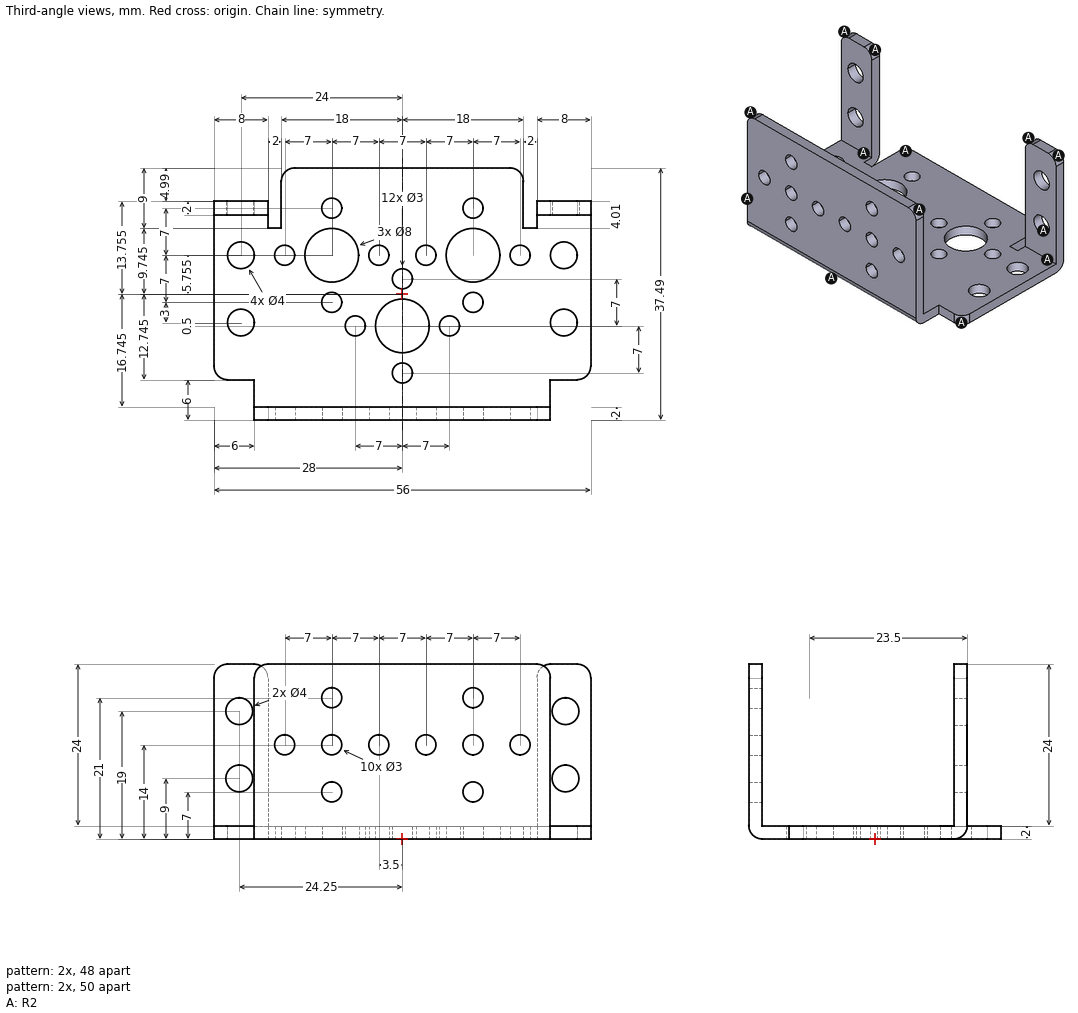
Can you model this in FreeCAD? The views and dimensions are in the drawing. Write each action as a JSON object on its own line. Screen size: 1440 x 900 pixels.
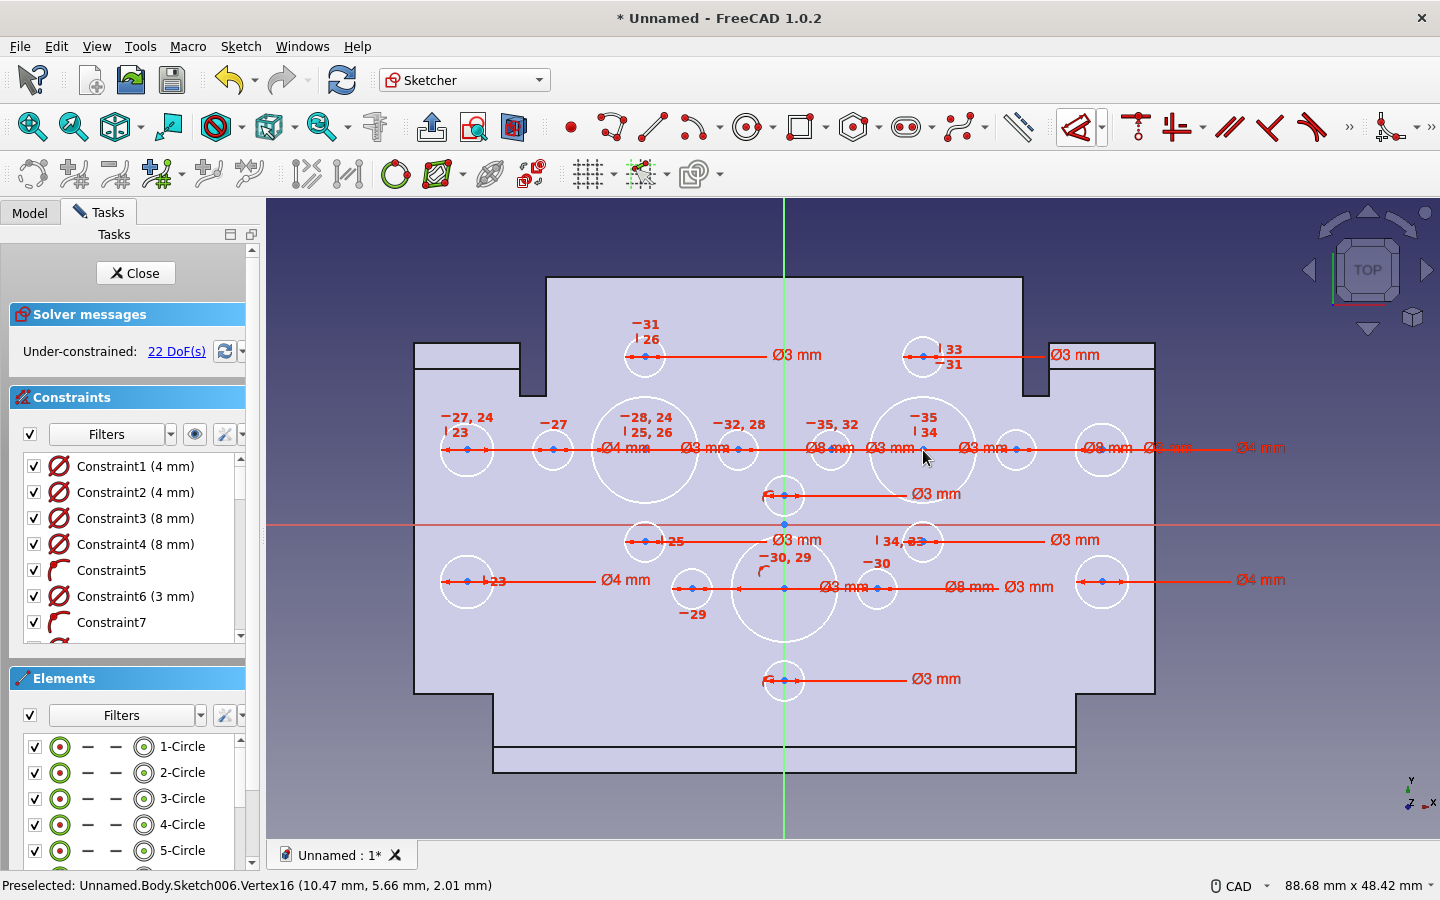
{"action": "left_click", "coordinate": [923, 450]}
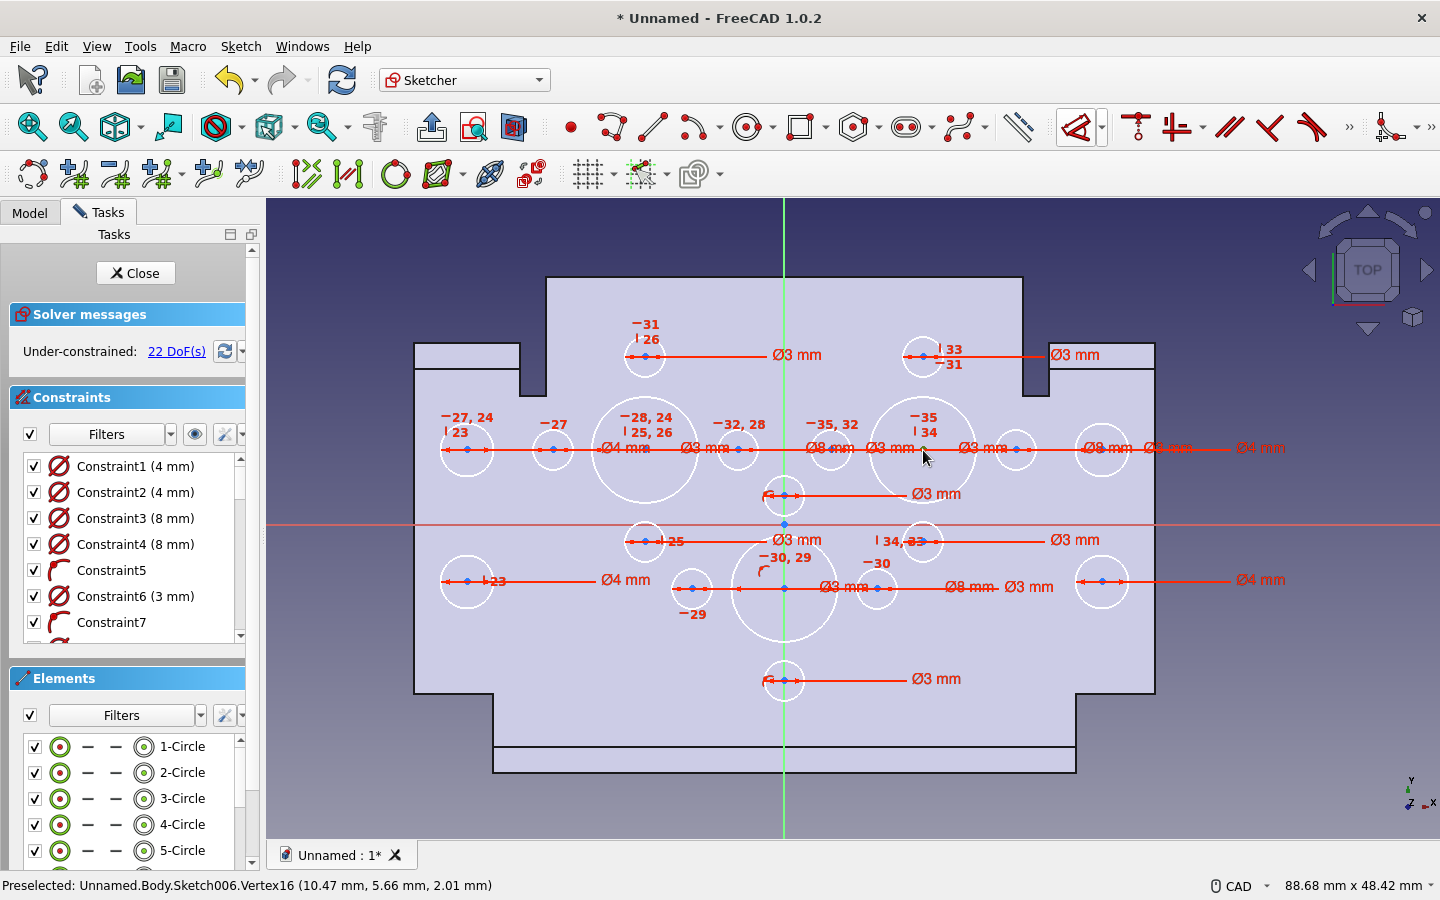
{"action": "left_click", "coordinate": [1016, 450]}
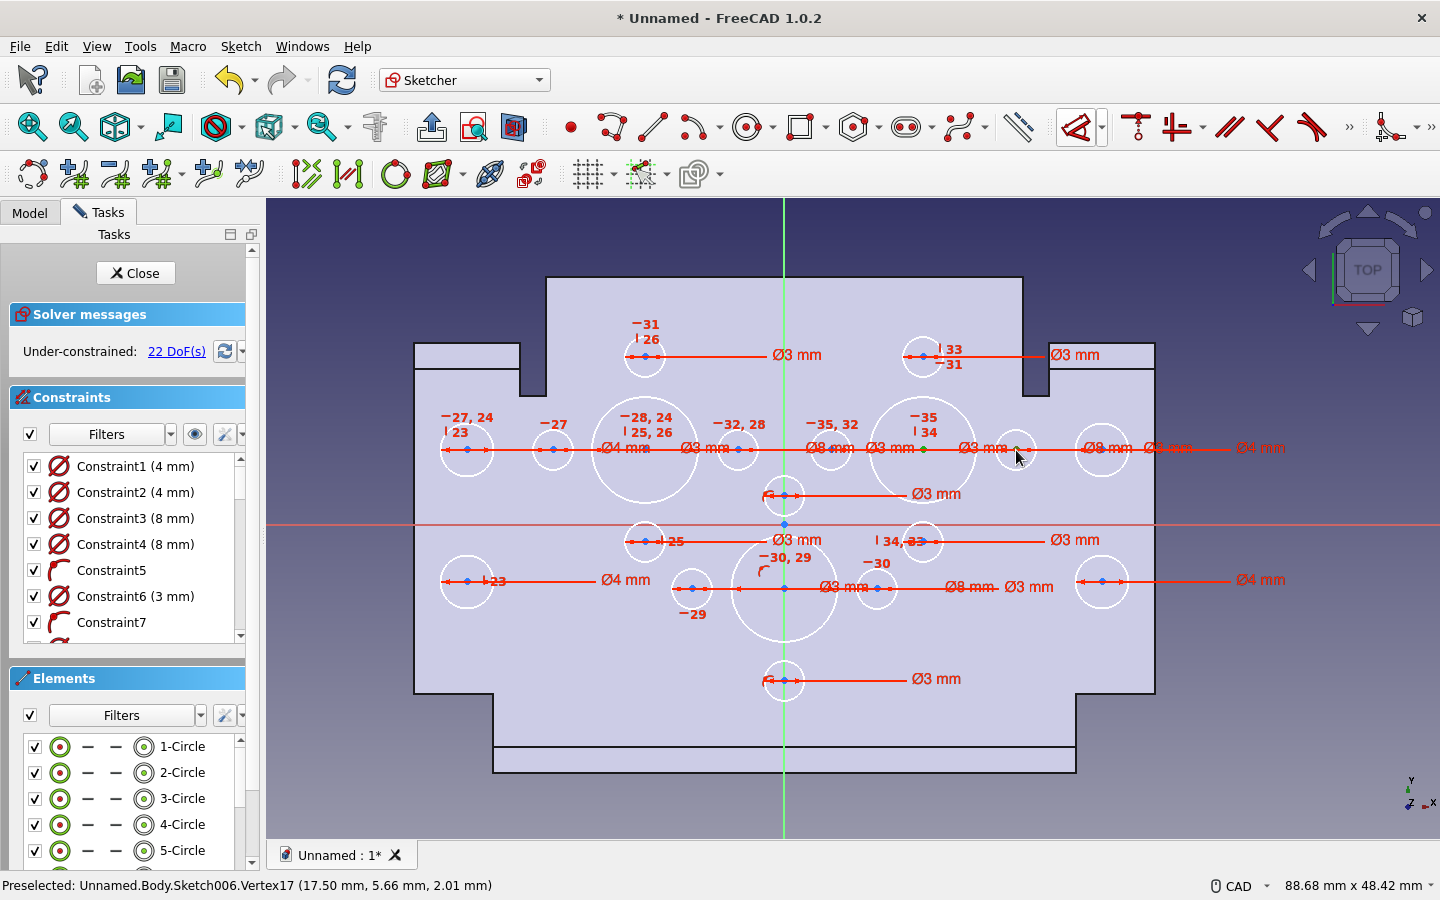
{"action": "key", "text": "h"}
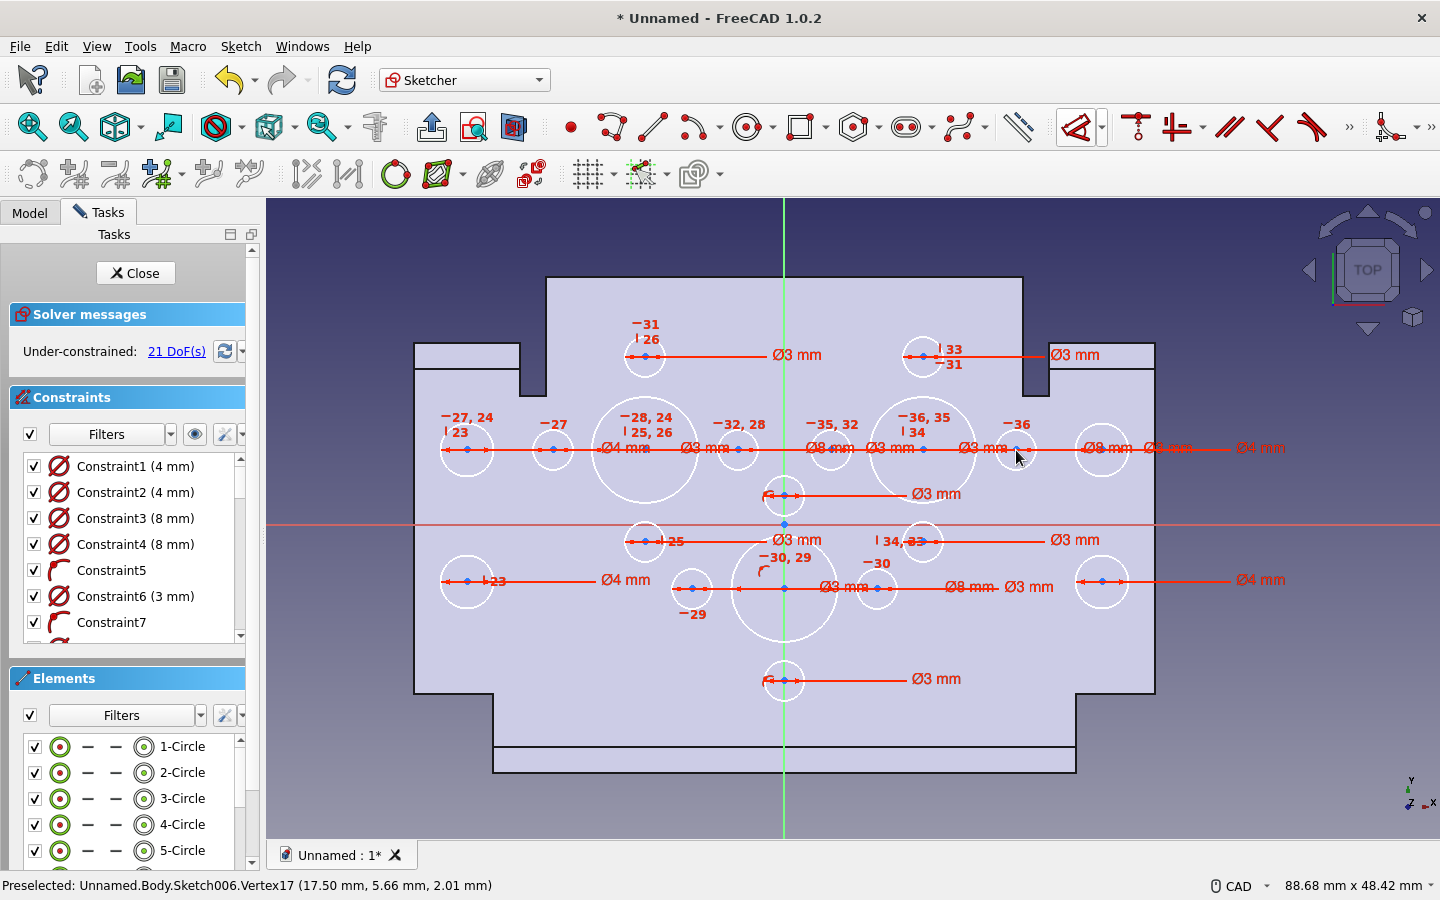
{"action": "left_click", "coordinate": [1102, 582]}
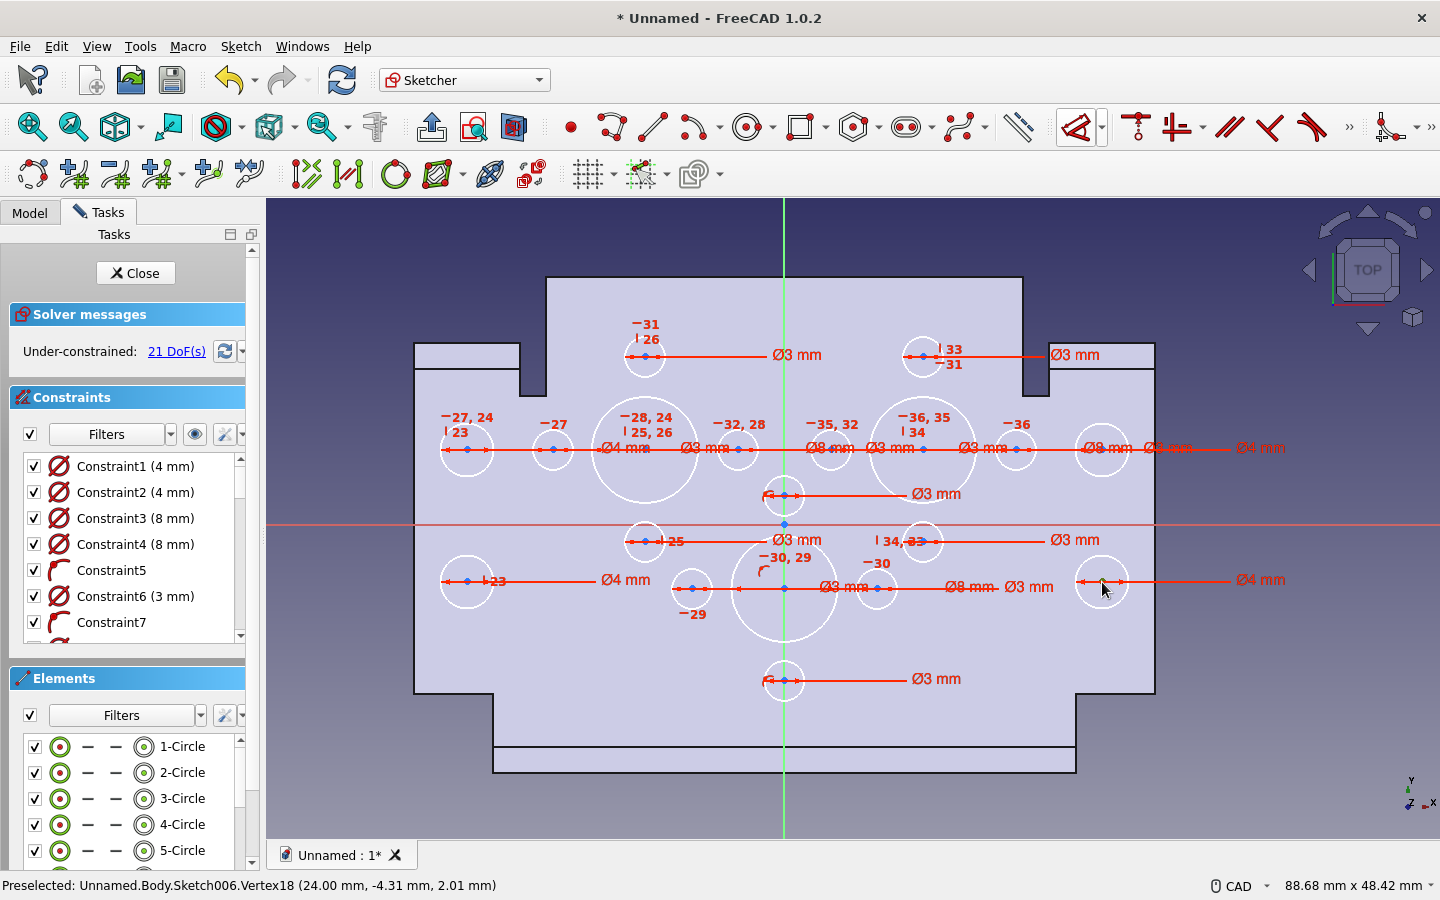
{"action": "left_click", "coordinate": [1102, 450]}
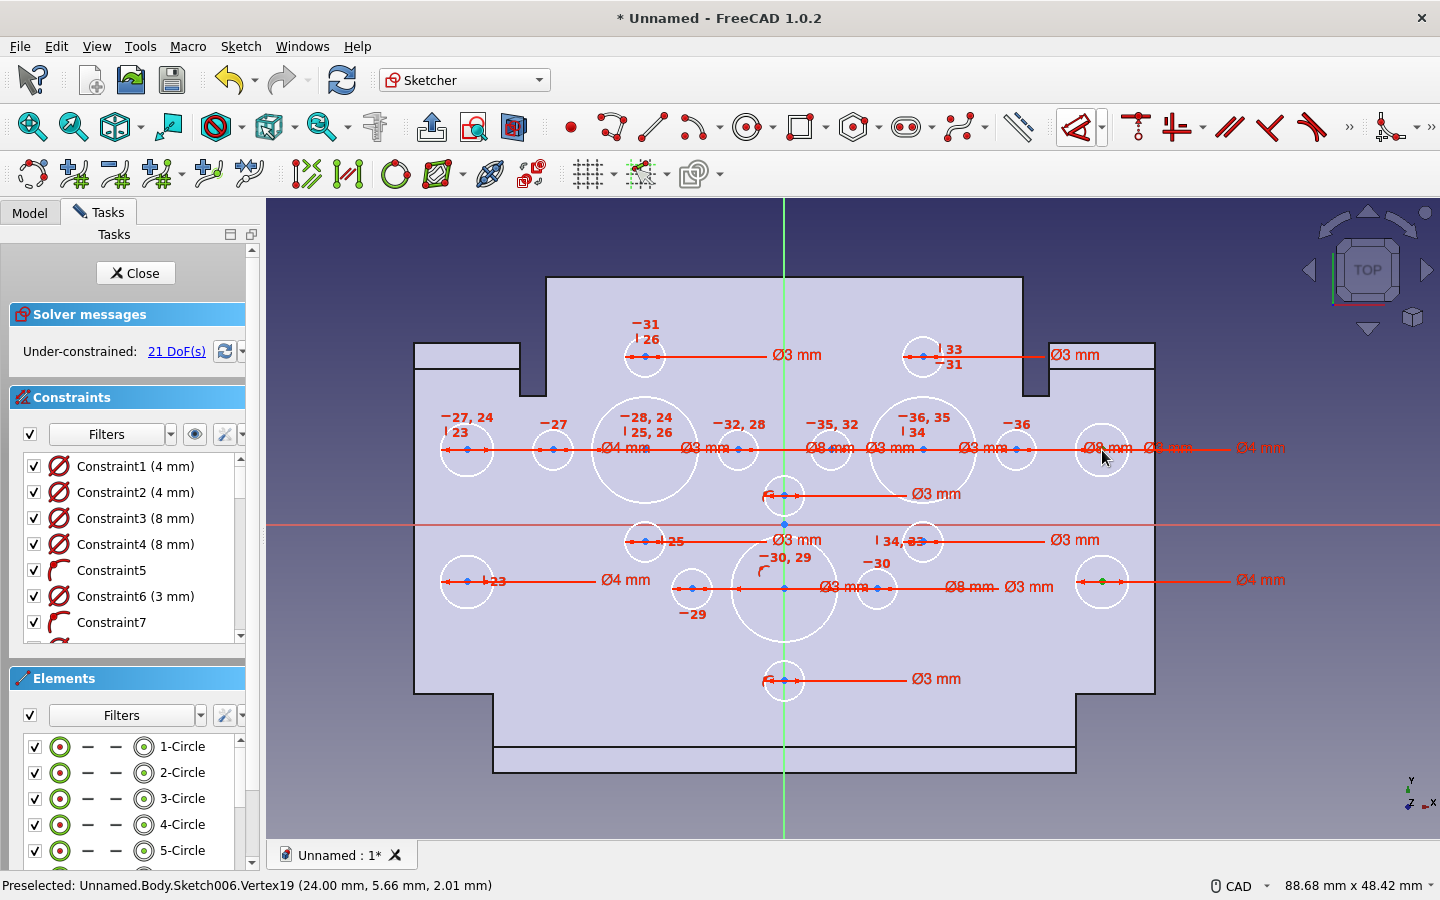
{"action": "left_click", "coordinate": [1202, 128]}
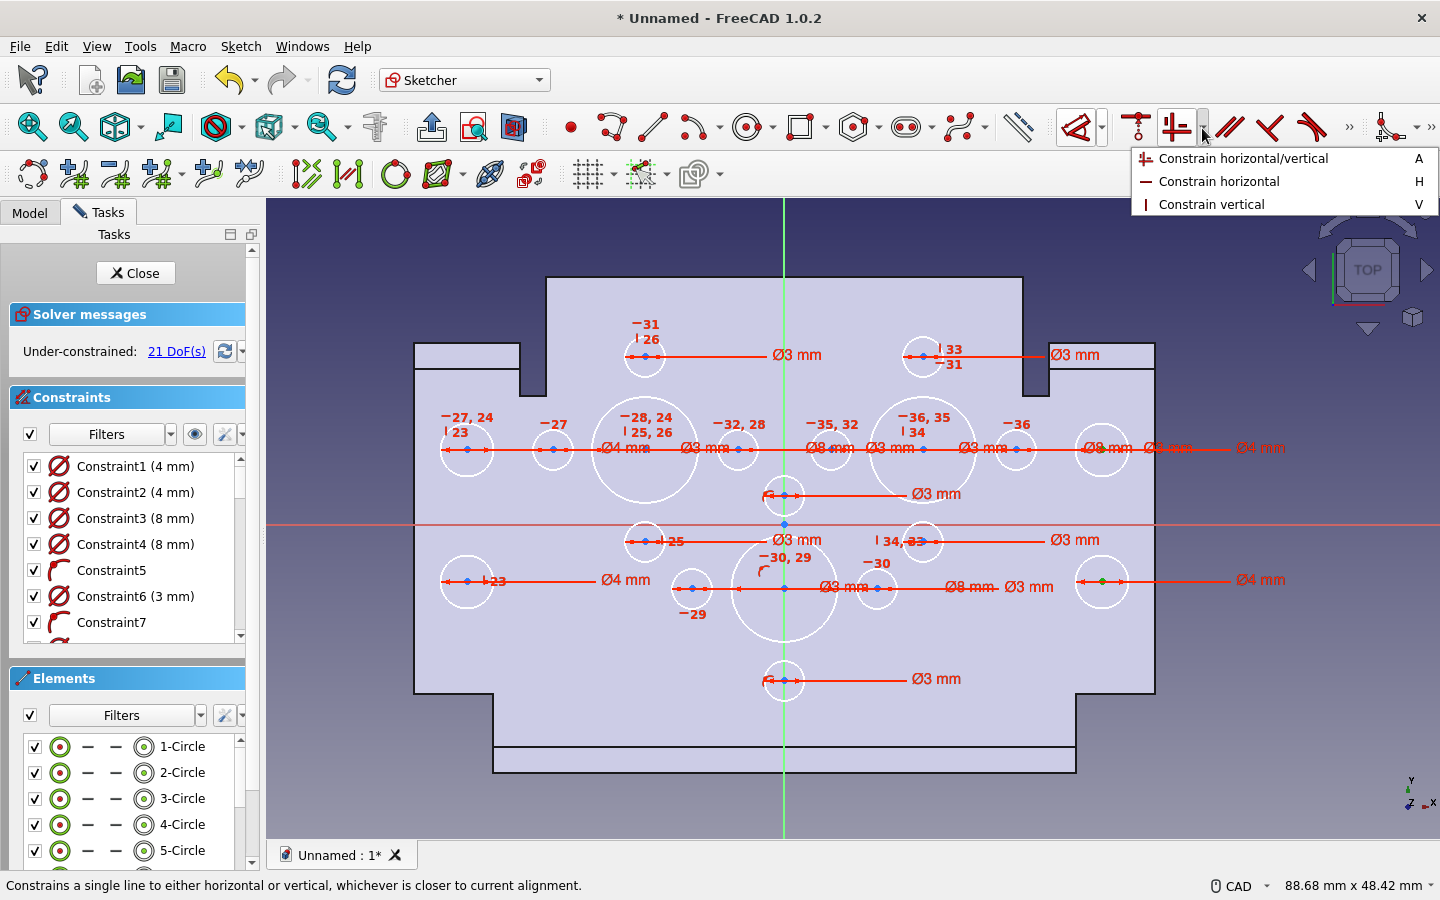
{"action": "left_click", "coordinate": [1285, 204]}